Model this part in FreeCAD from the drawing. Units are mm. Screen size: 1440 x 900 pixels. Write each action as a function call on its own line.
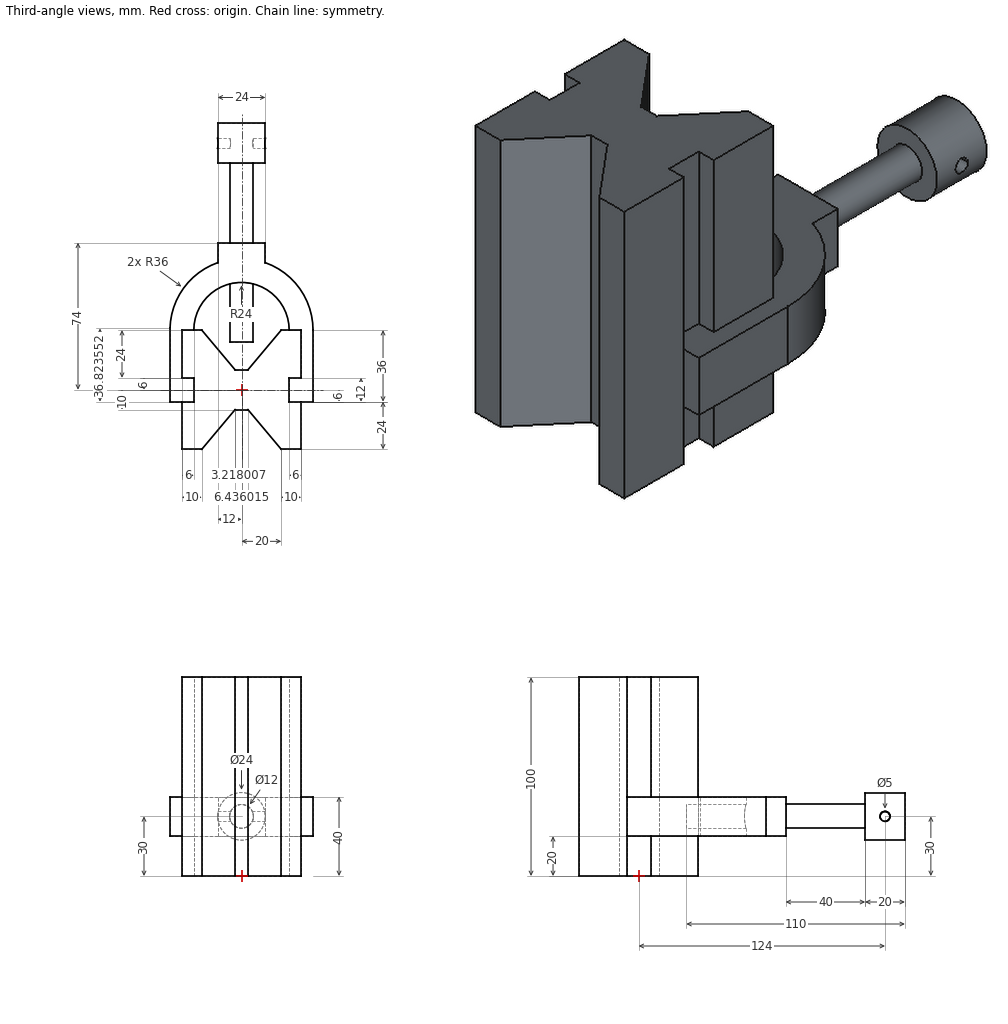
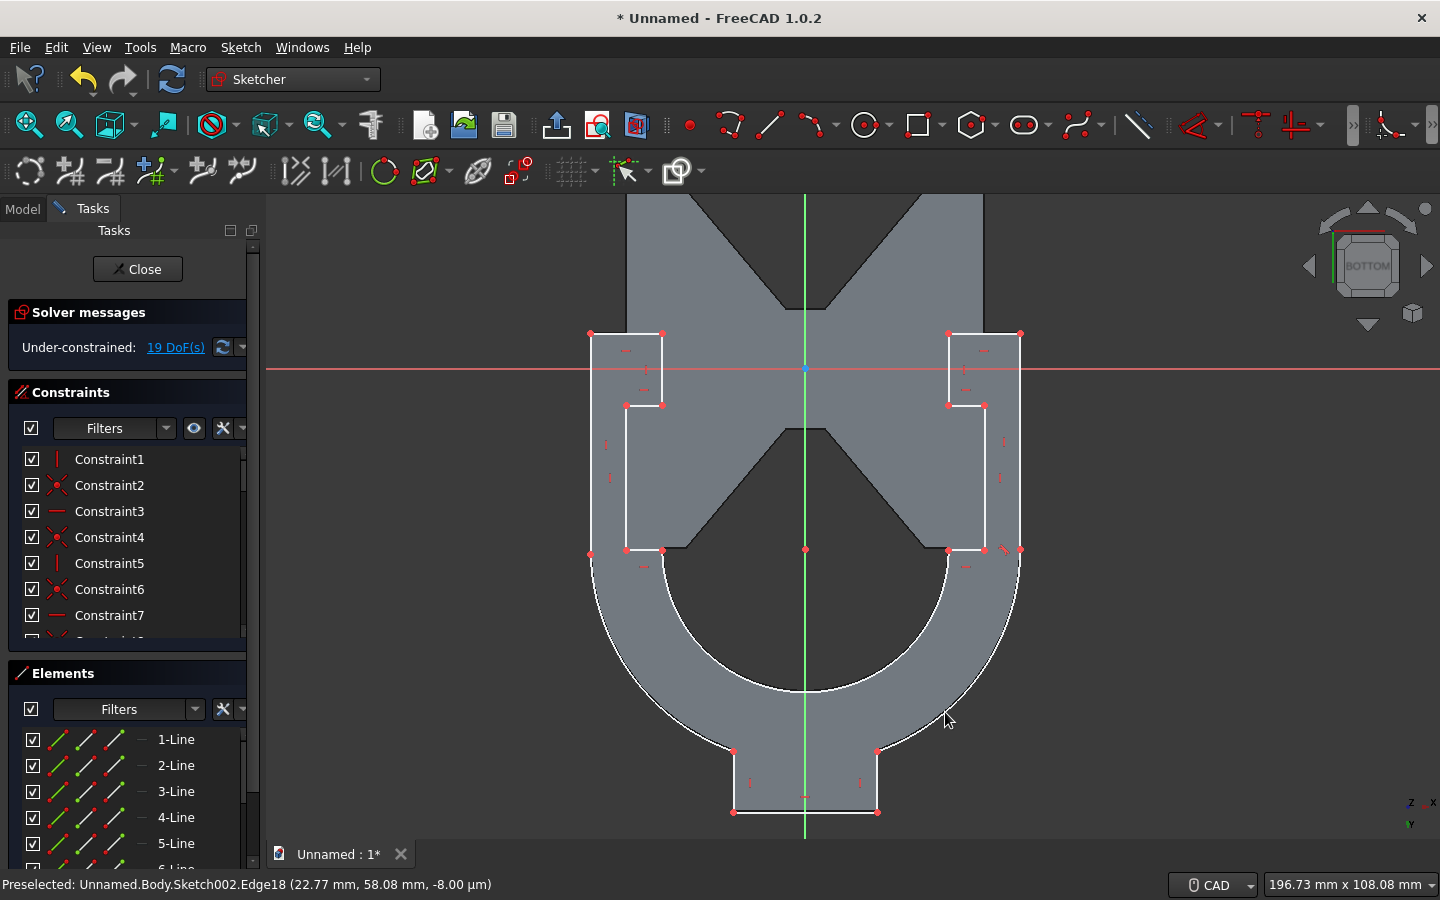
click(607, 630)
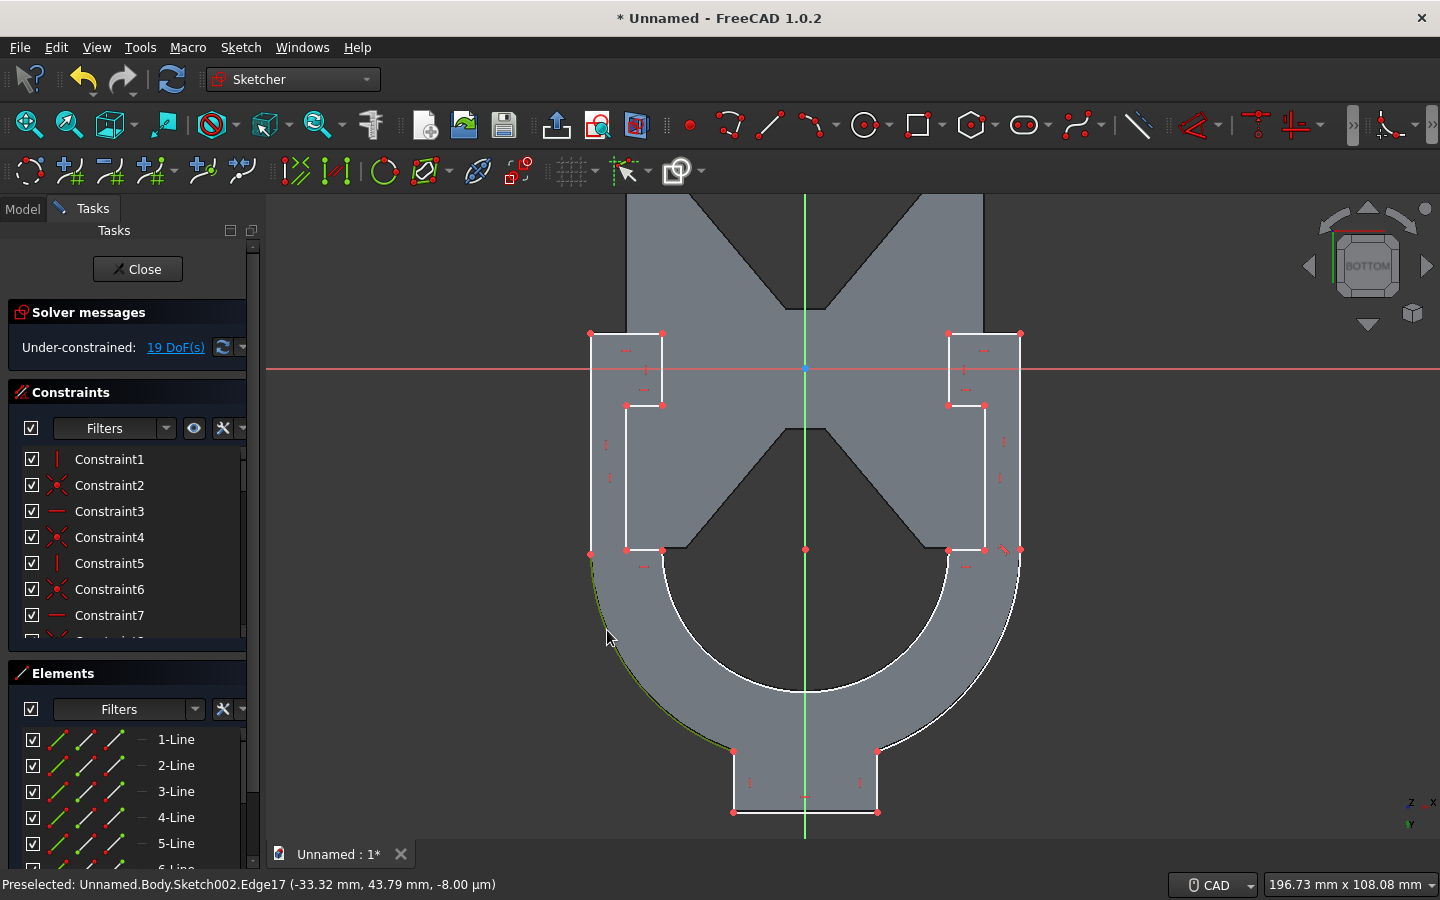
click(945, 712)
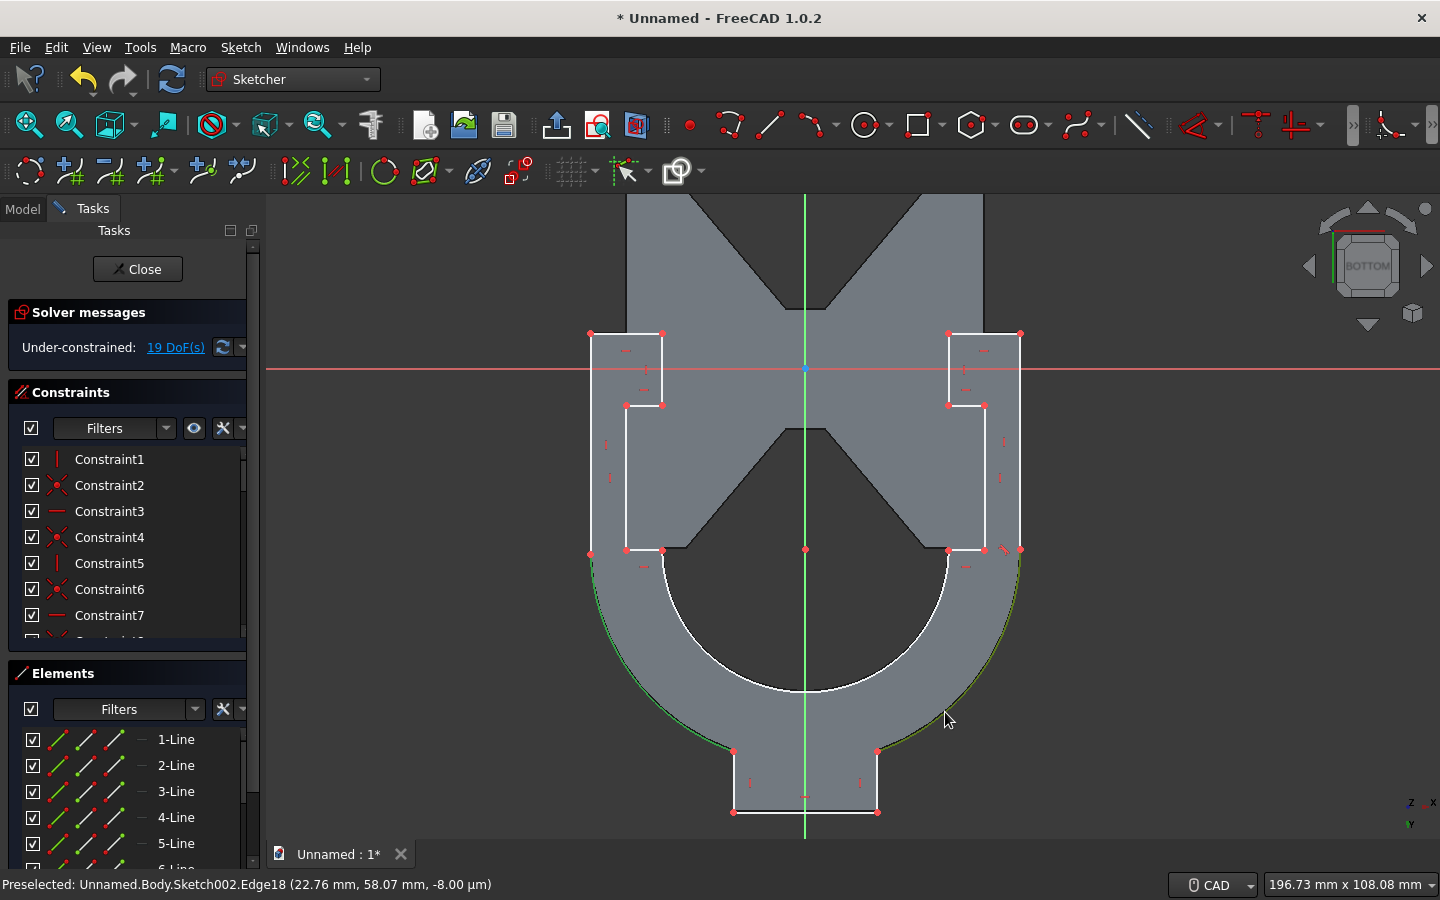
key(e)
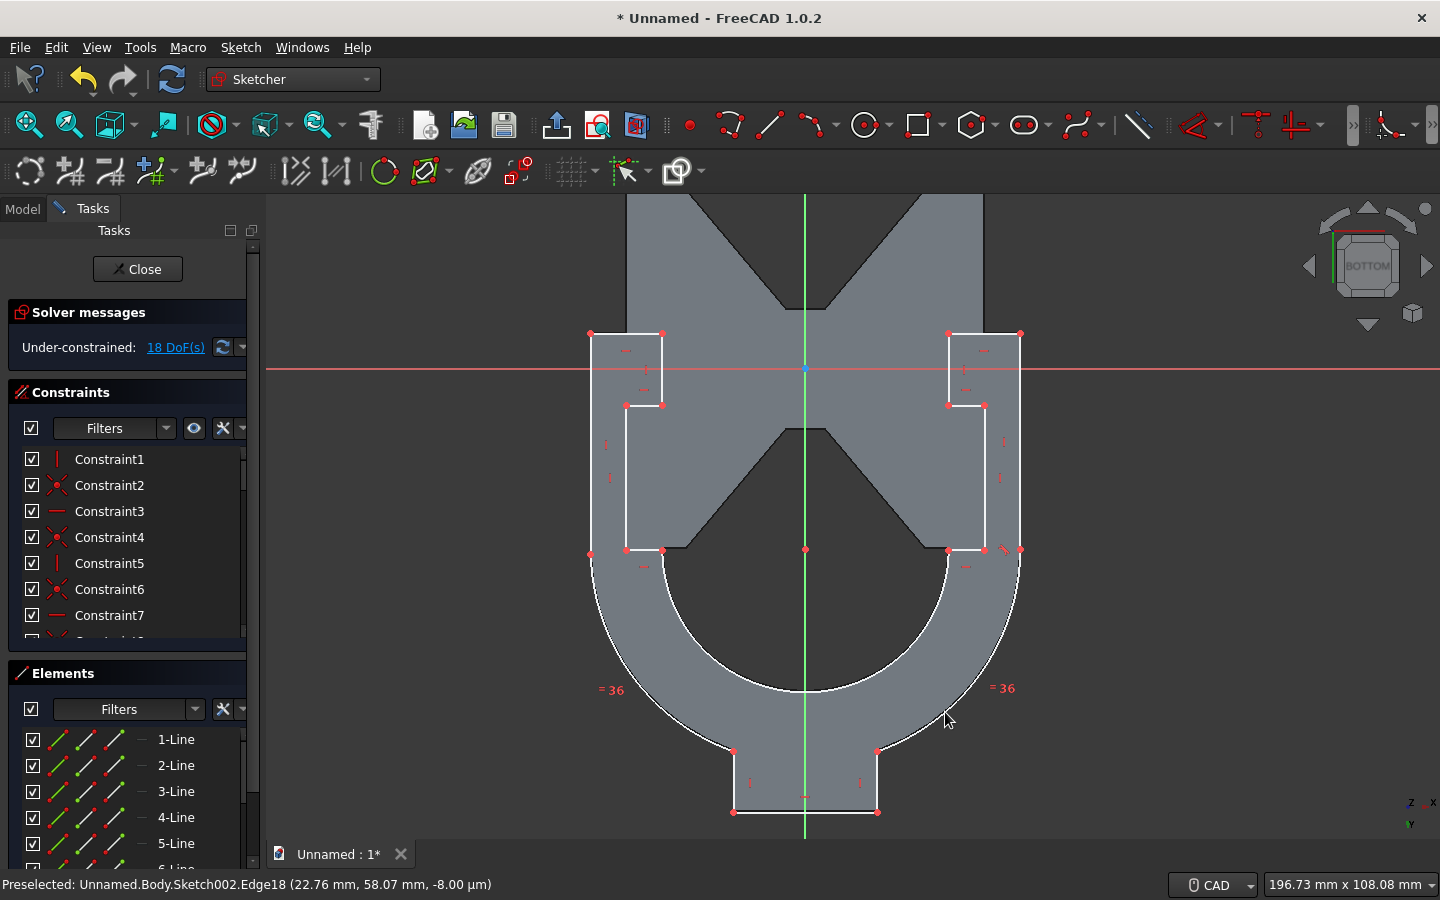
click(805, 549)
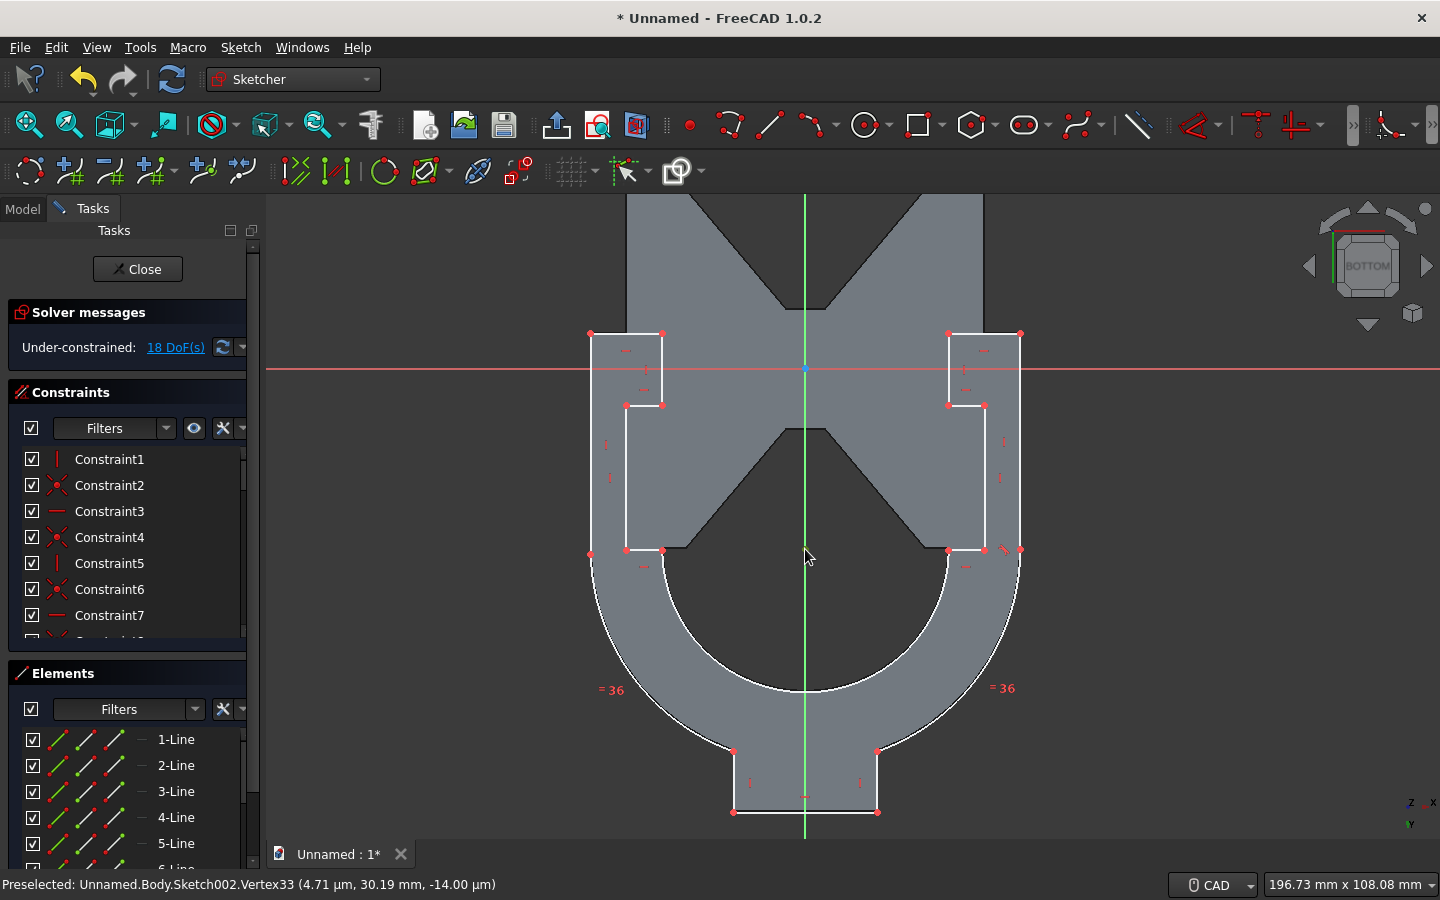
click(805, 769)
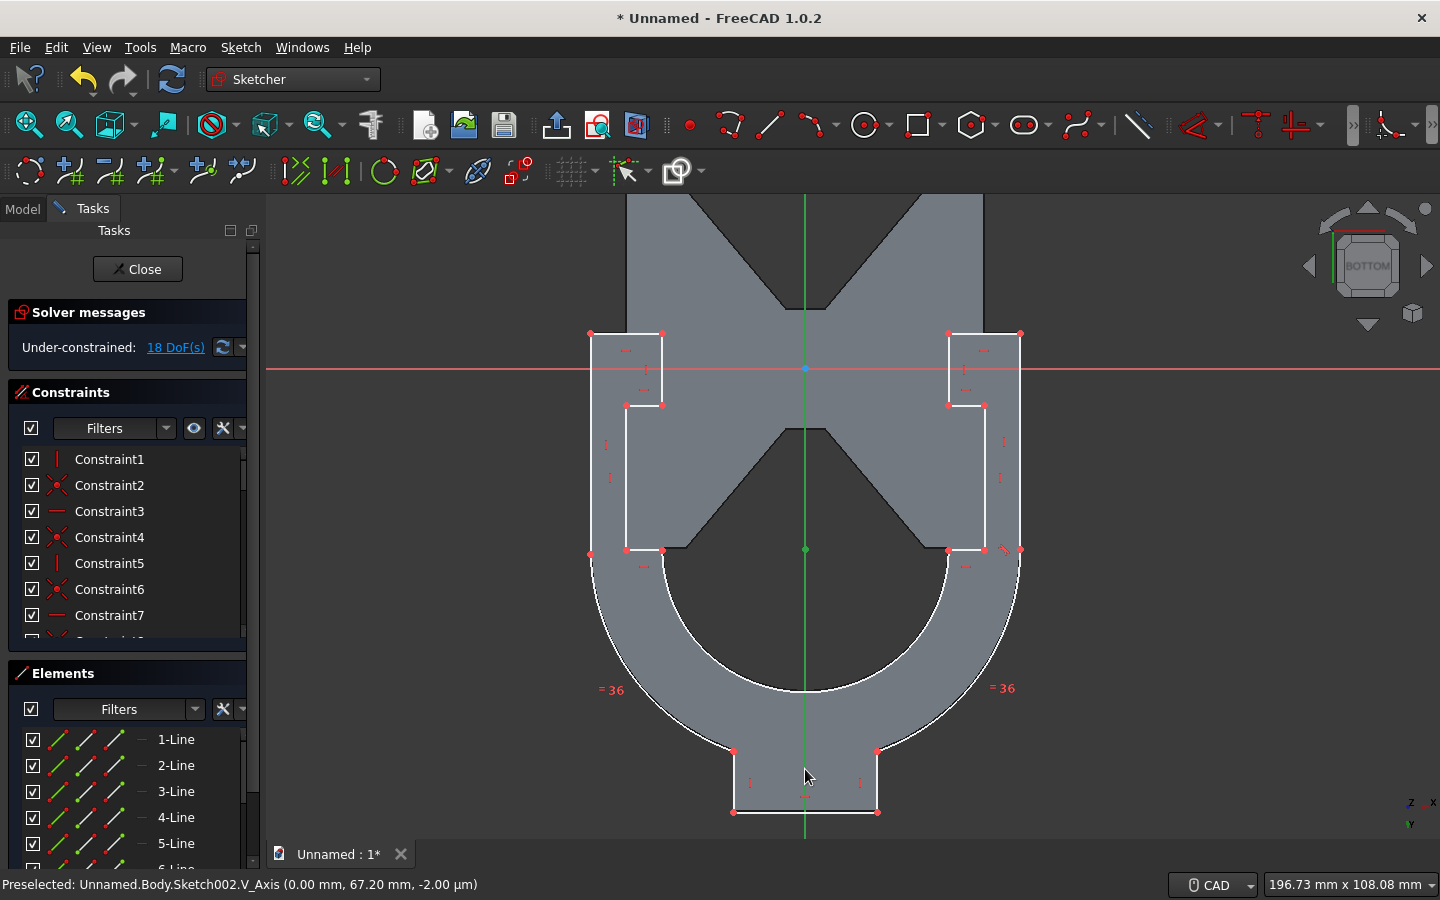
click(1256, 126)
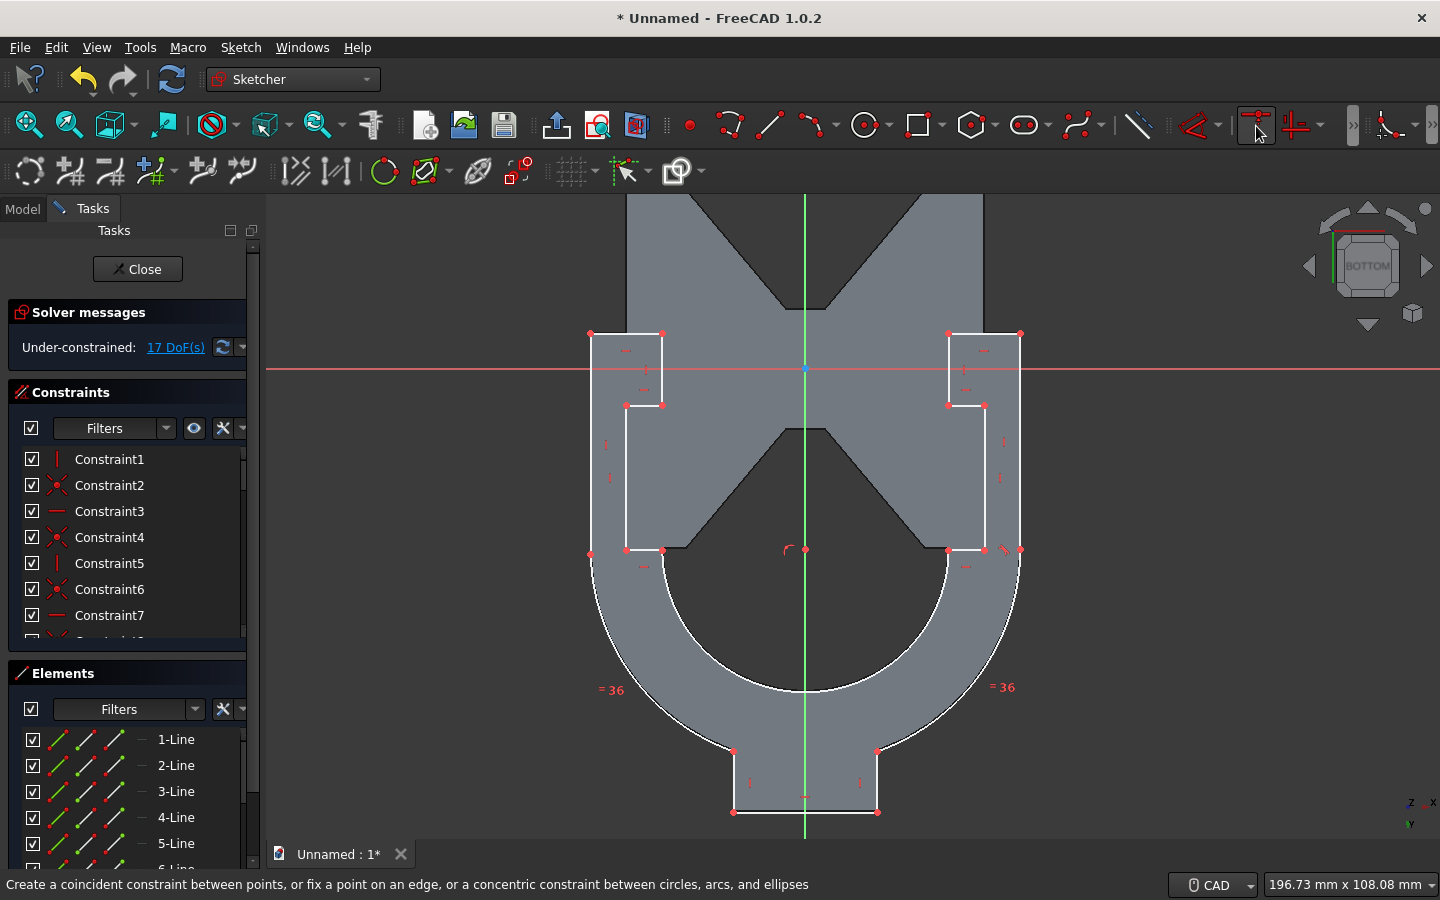
click(985, 550)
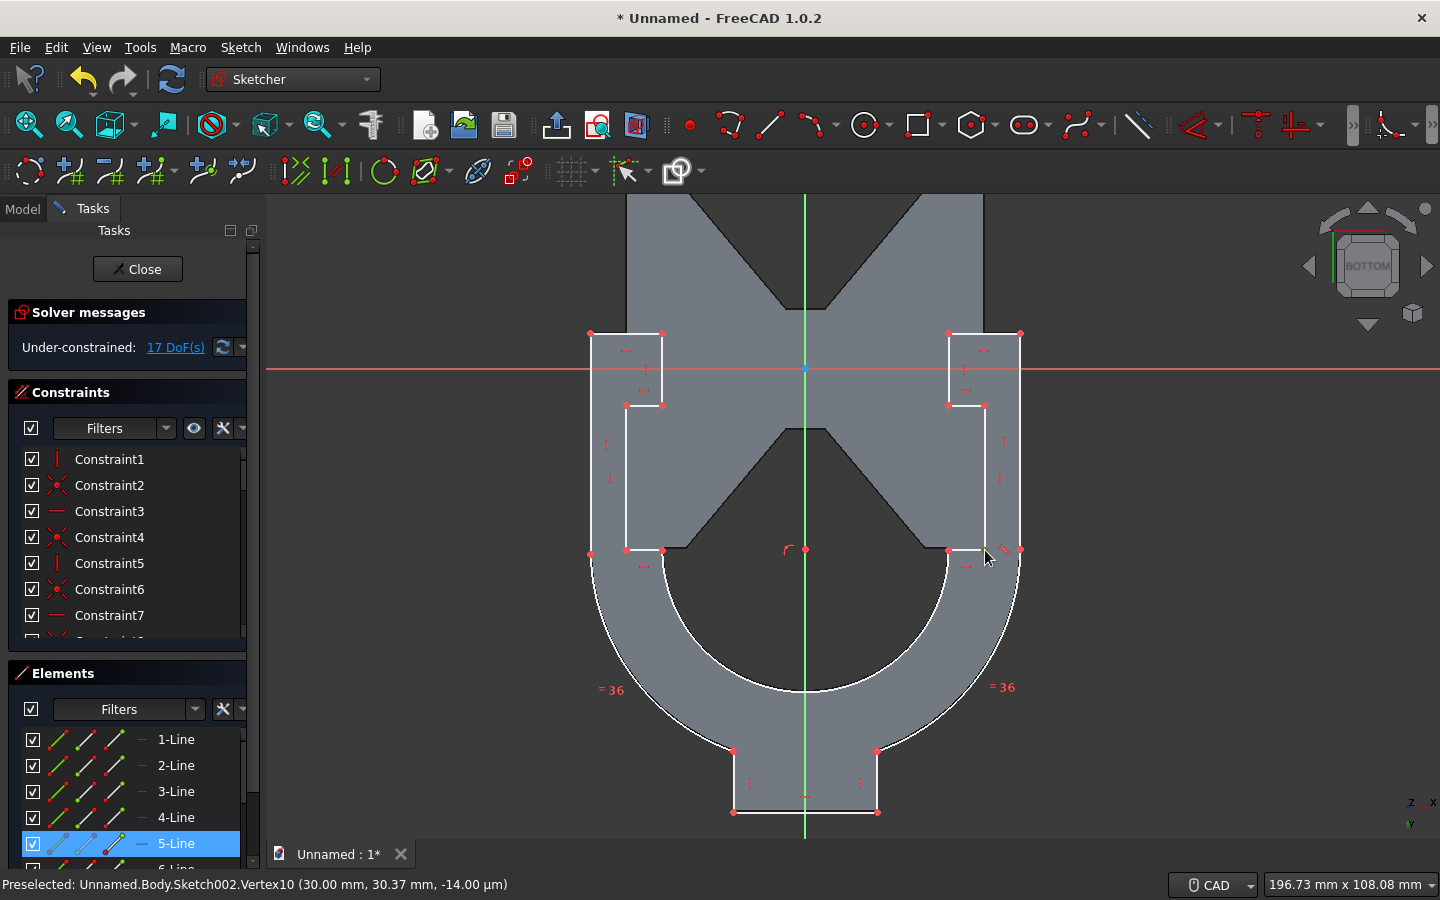
click(626, 550)